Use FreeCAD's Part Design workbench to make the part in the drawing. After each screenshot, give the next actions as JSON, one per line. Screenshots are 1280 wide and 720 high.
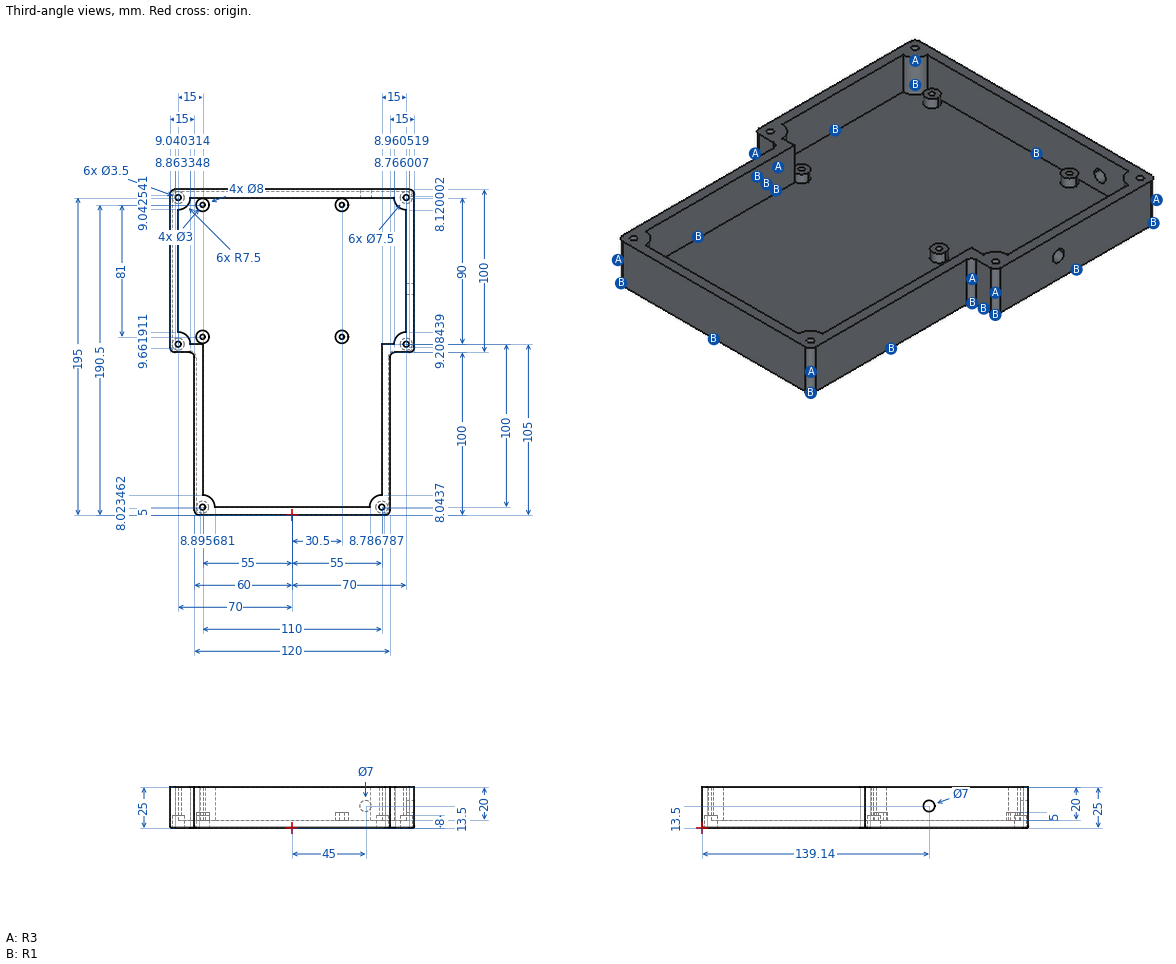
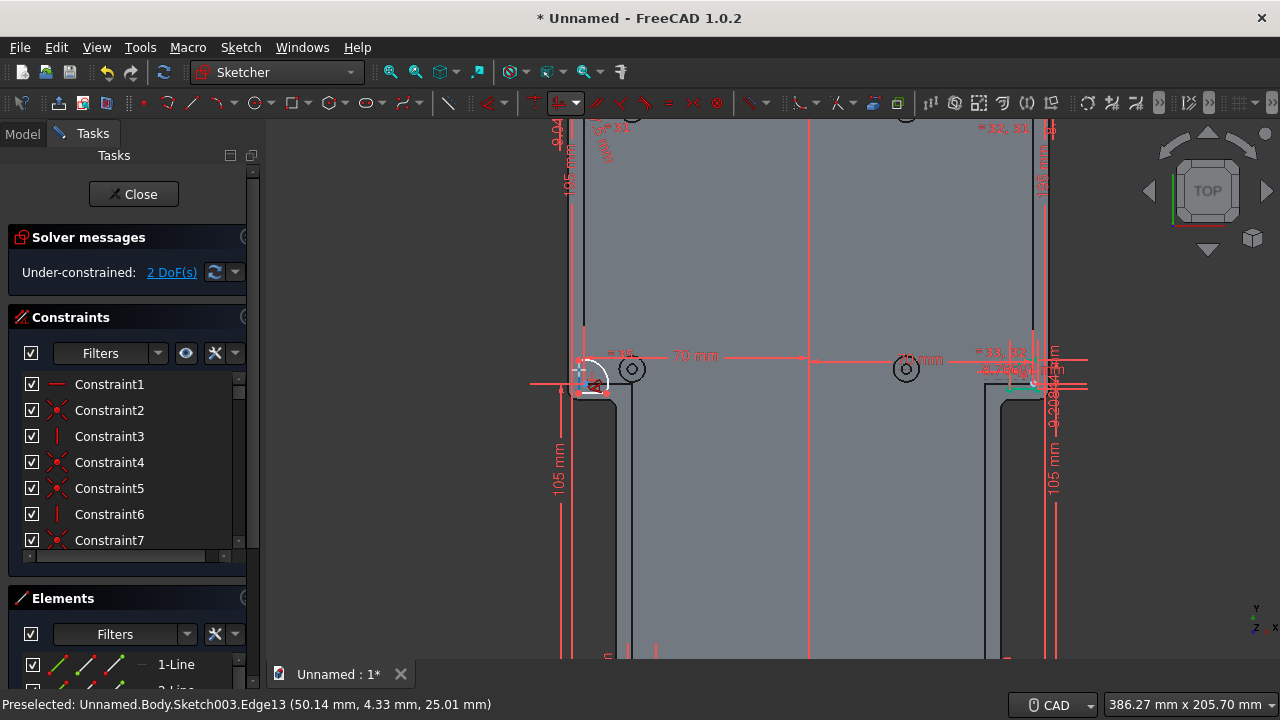
{"action": "left_click", "coordinate": [578, 370]}
{"action": "left_click", "coordinate": [544, 380]}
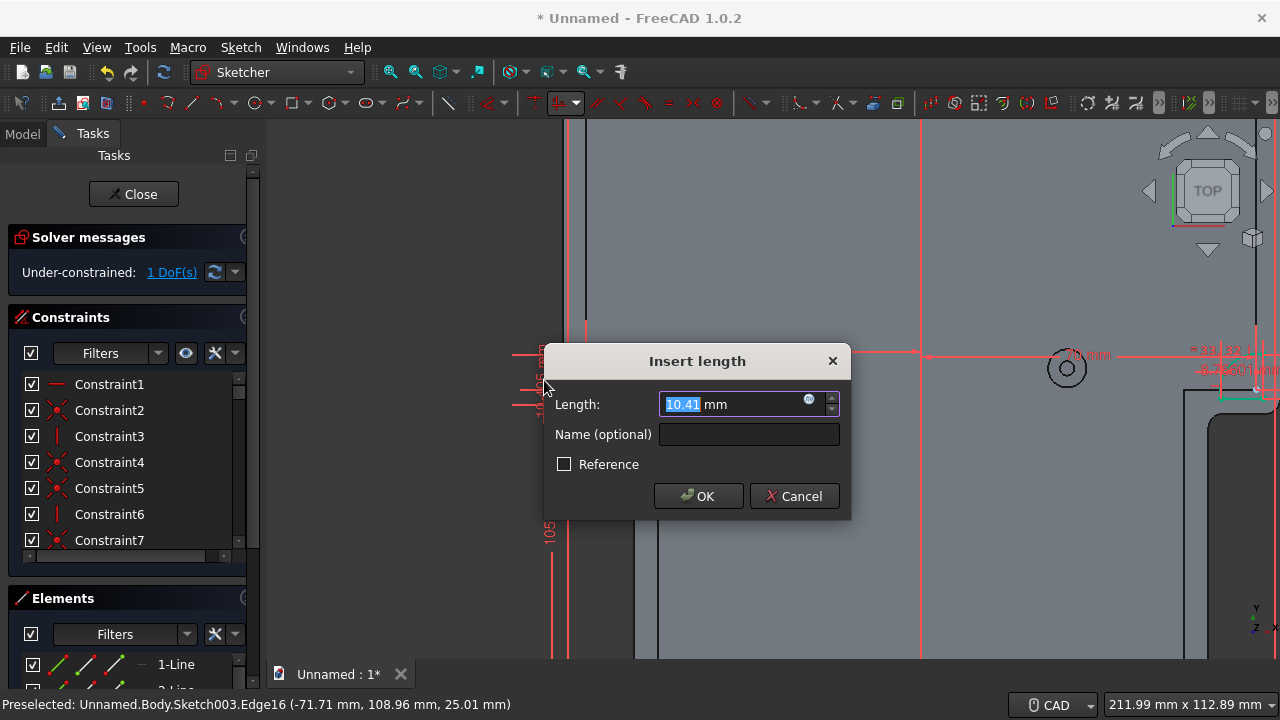
{"action": "type", "text": "9.661911"}
{"action": "key", "text": "Return"}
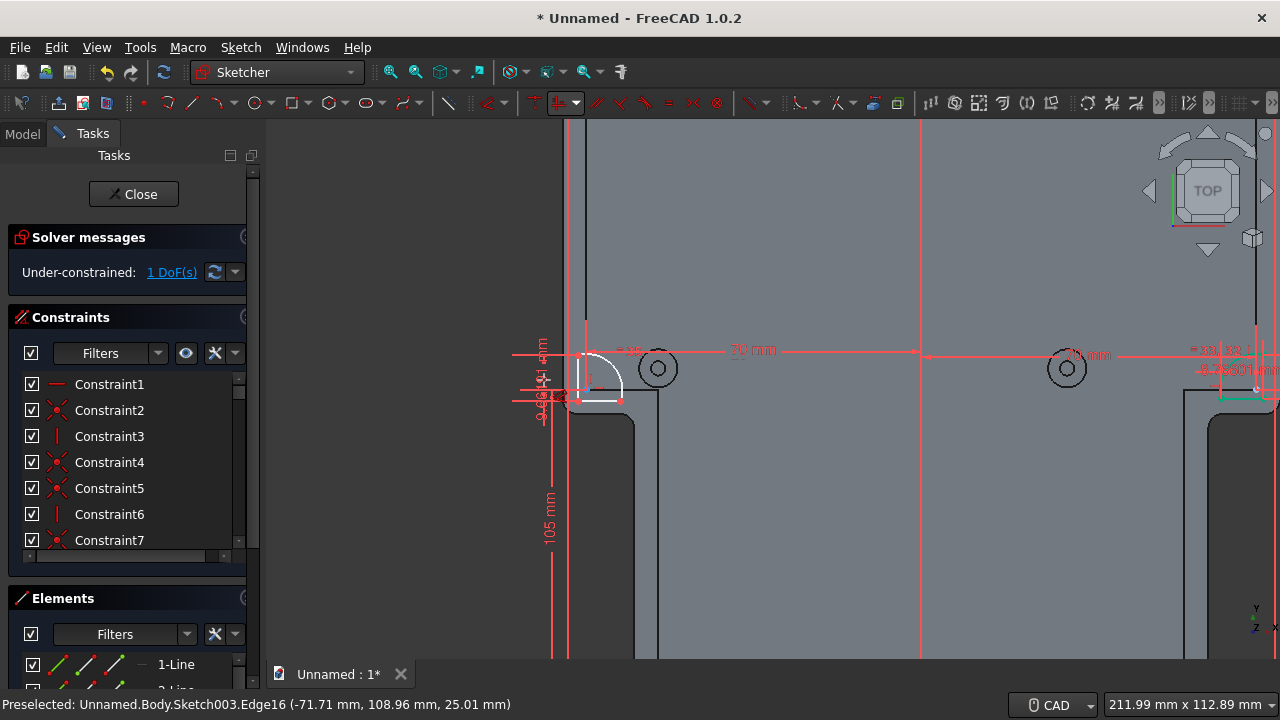
{"action": "left_click", "coordinate": [591, 401]}
{"action": "left_click", "coordinate": [599, 435]}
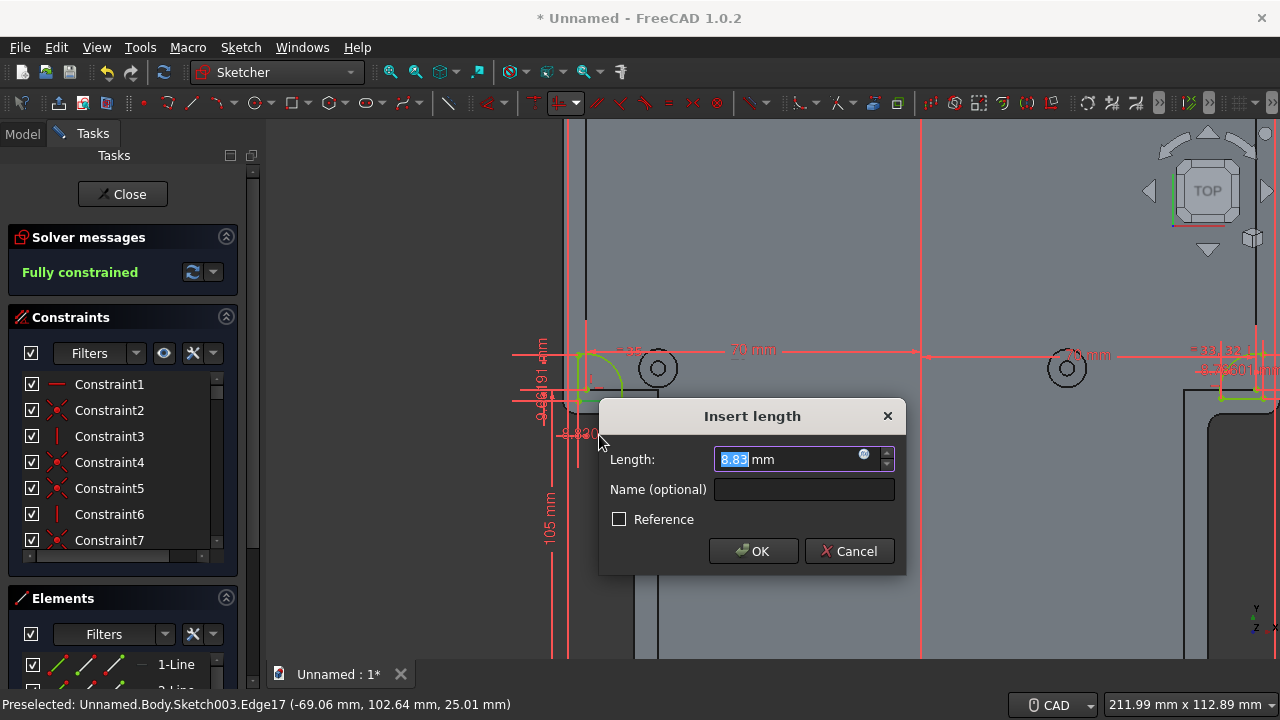
{"action": "type", "text": "8.863348"}
{"action": "key", "text": "Return"}
{"action": "key", "text": "Escape"}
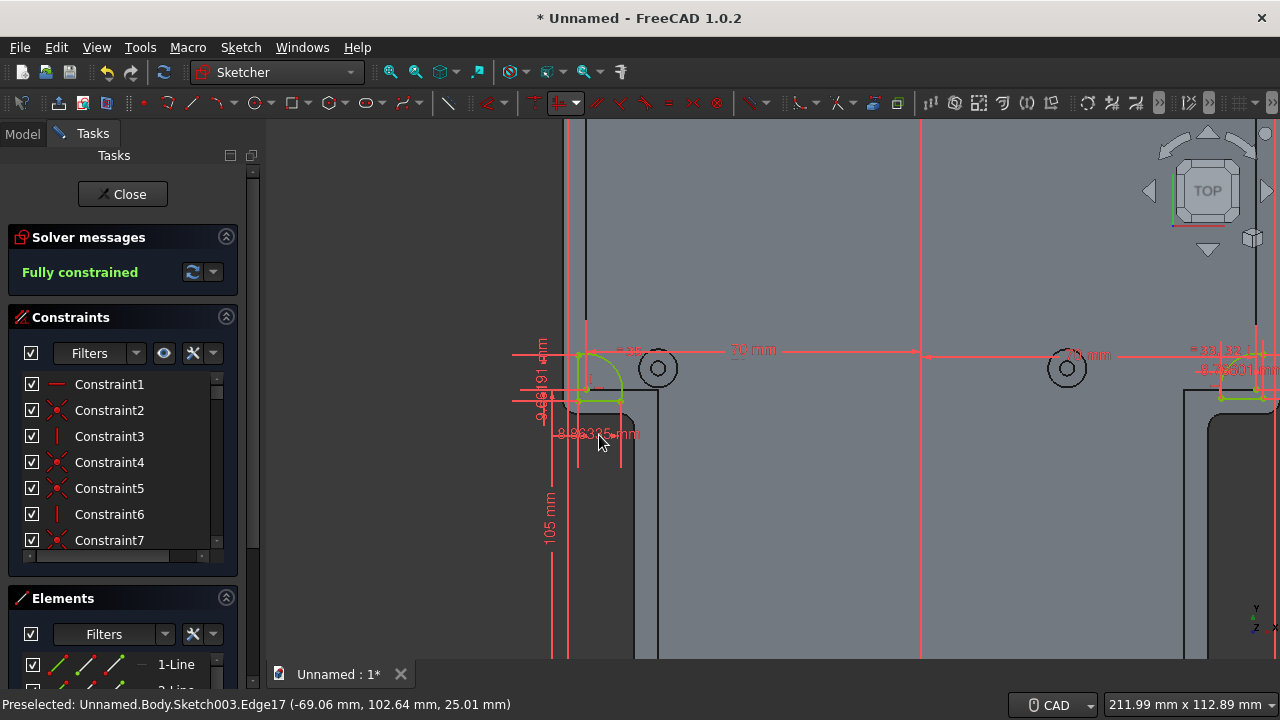
{"action": "left_click", "coordinate": [123, 194]}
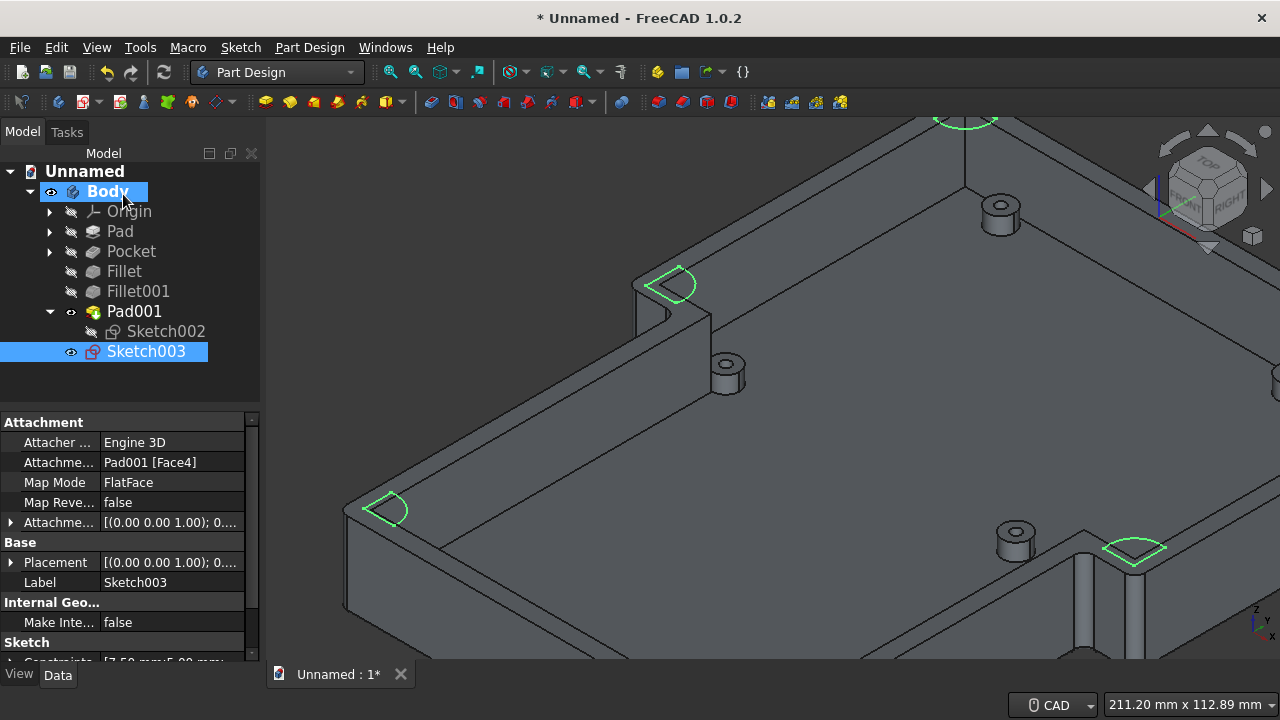
{"action": "left_click", "coordinate": [266, 102]}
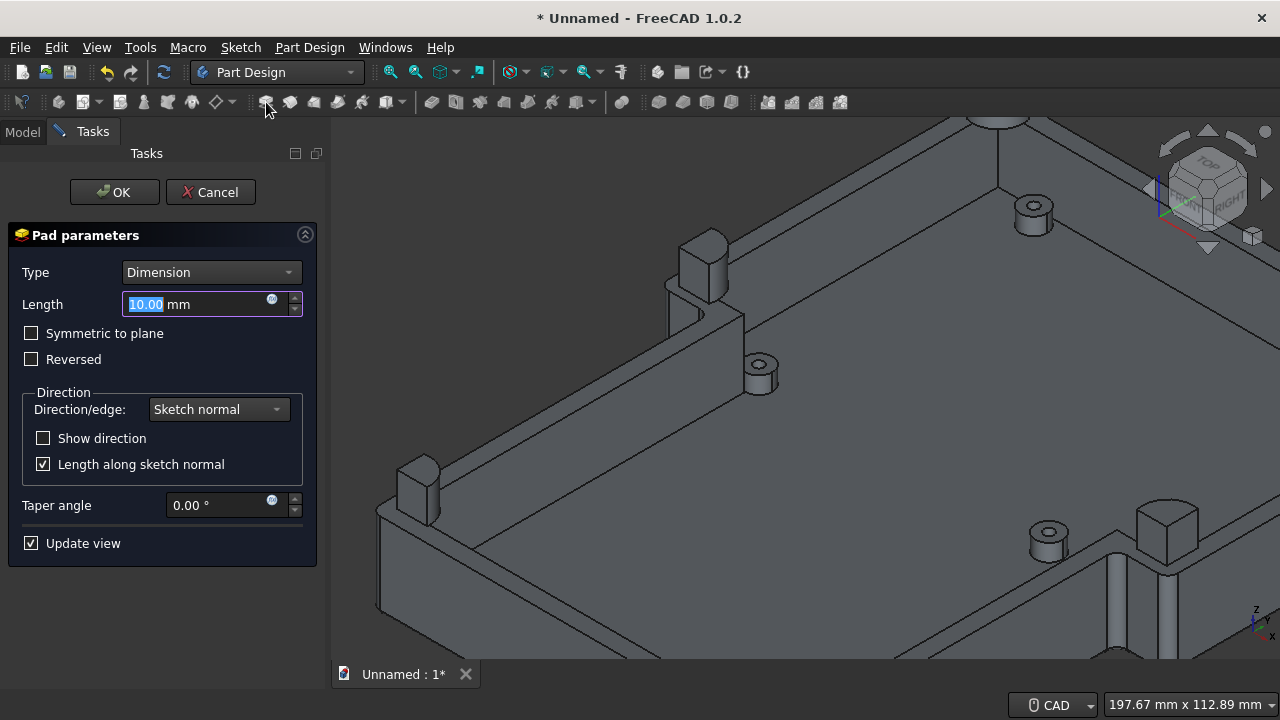
{"action": "type", "text": "25"}
{"action": "key", "text": "Tab"}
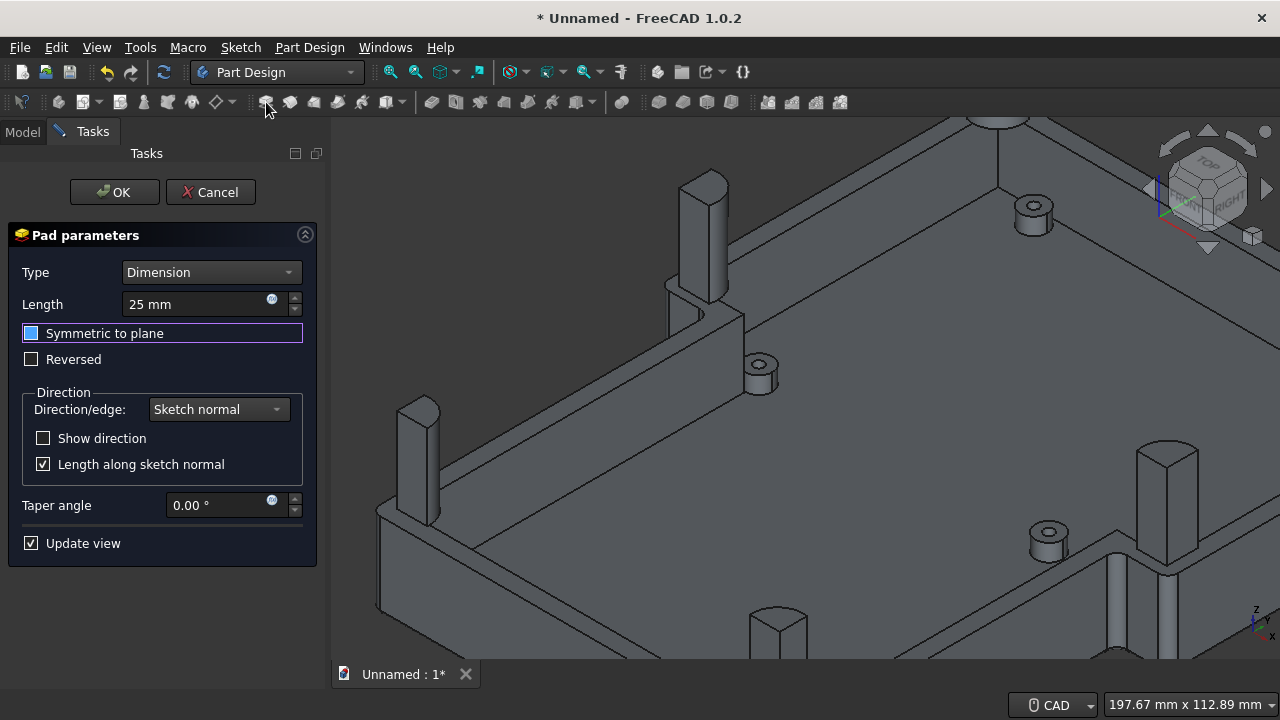
{"action": "left_click", "coordinate": [30, 359]}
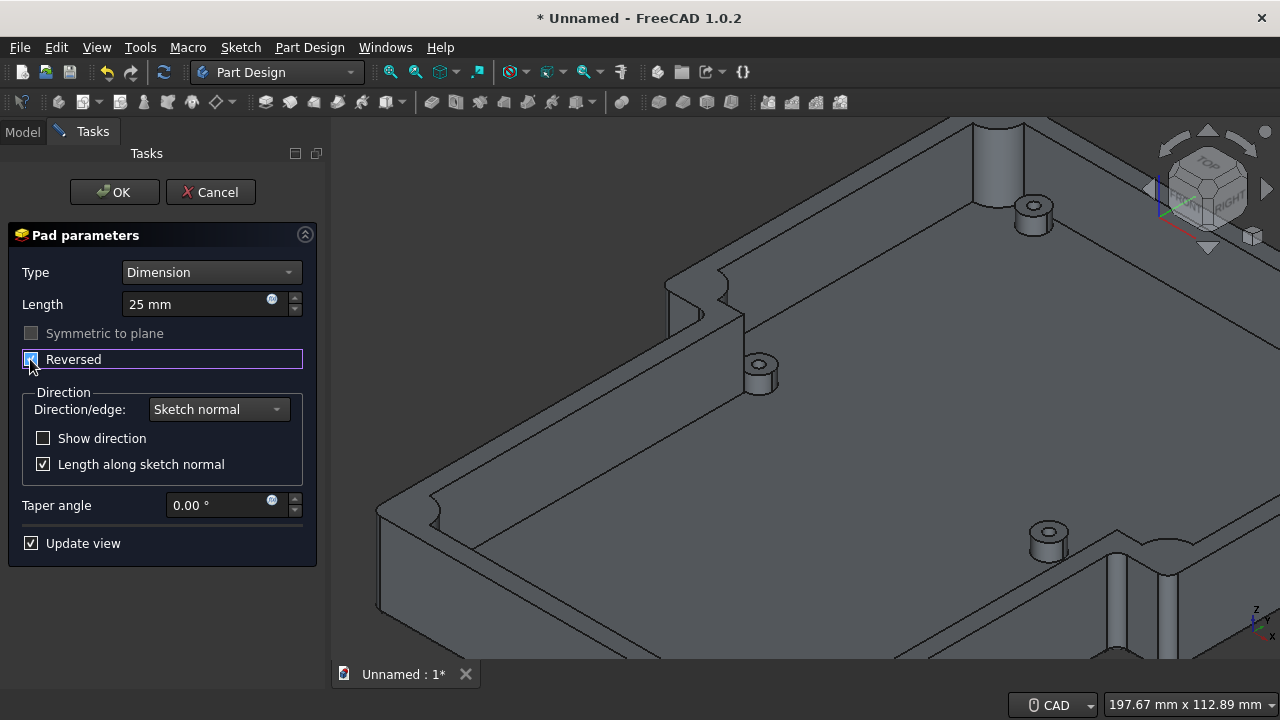
{"action": "left_click", "coordinate": [115, 192]}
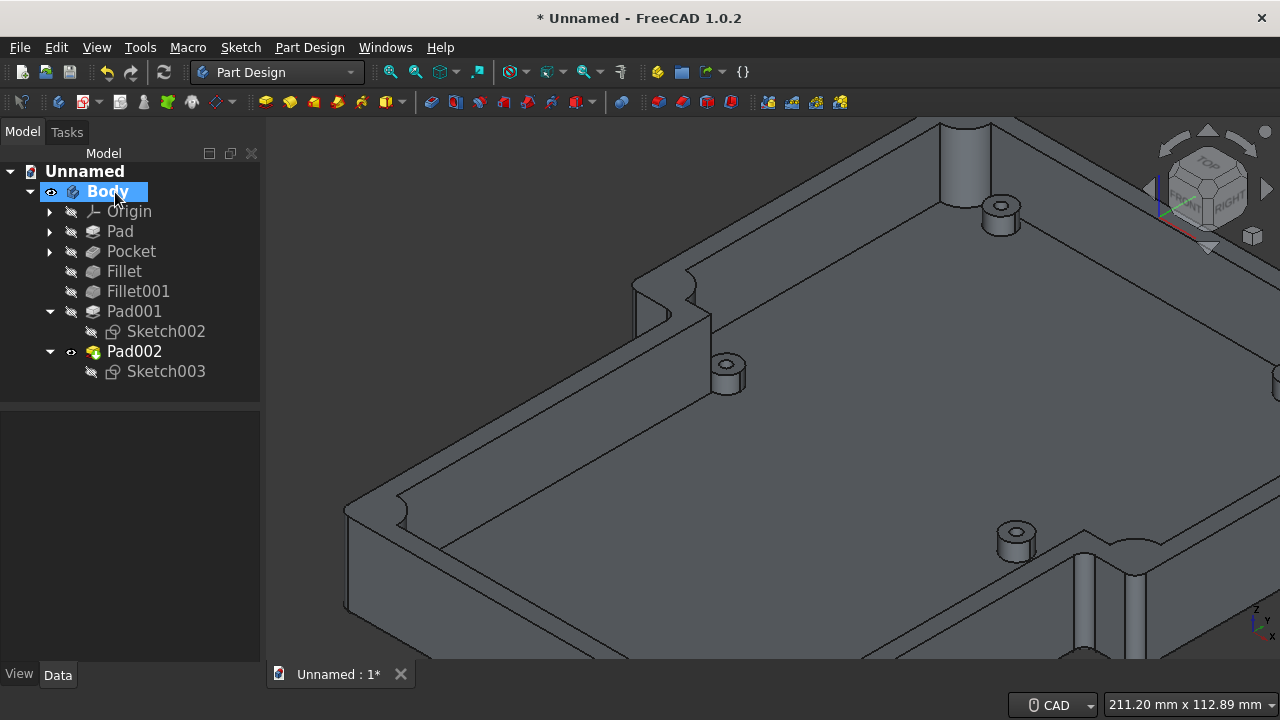
{"action": "key", "text": "v f"}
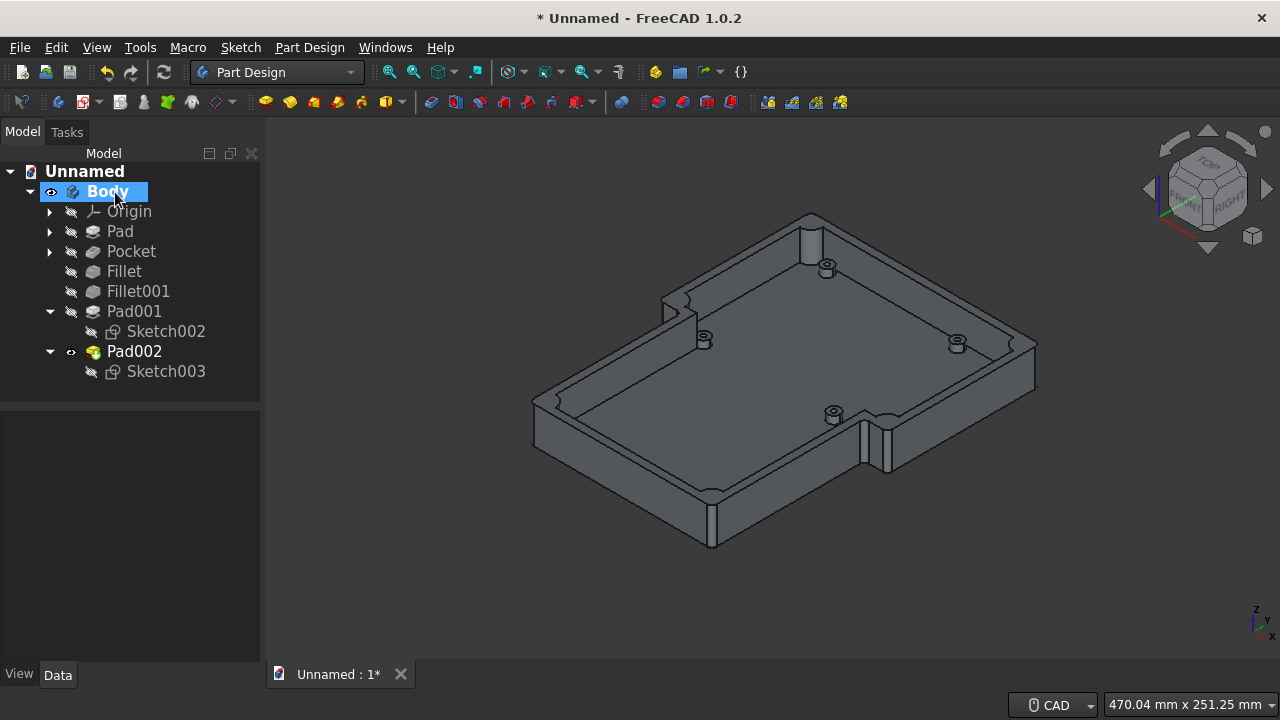
{"action": "left_click", "coordinate": [890, 418]}